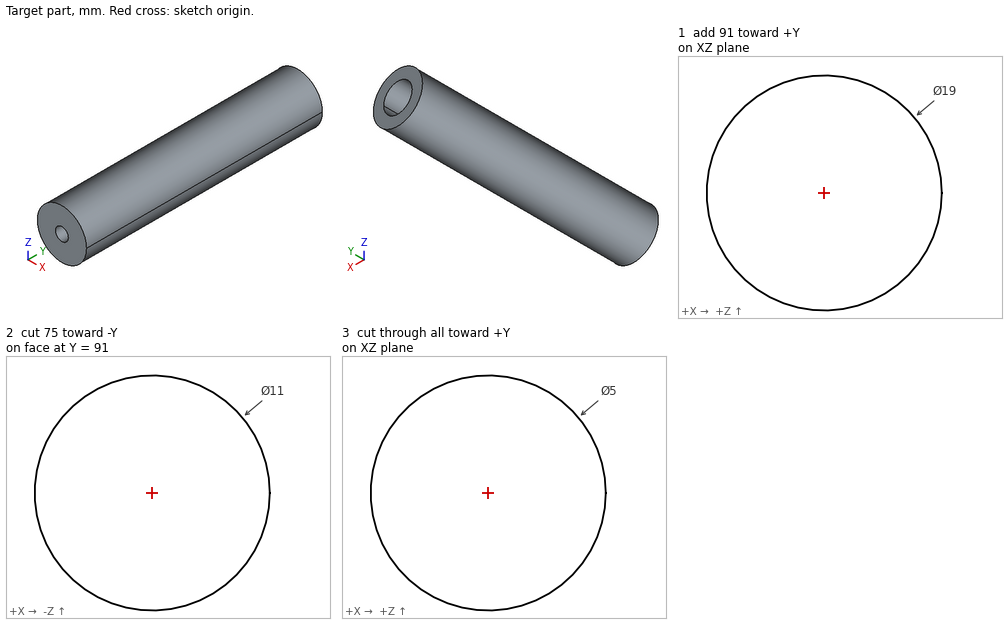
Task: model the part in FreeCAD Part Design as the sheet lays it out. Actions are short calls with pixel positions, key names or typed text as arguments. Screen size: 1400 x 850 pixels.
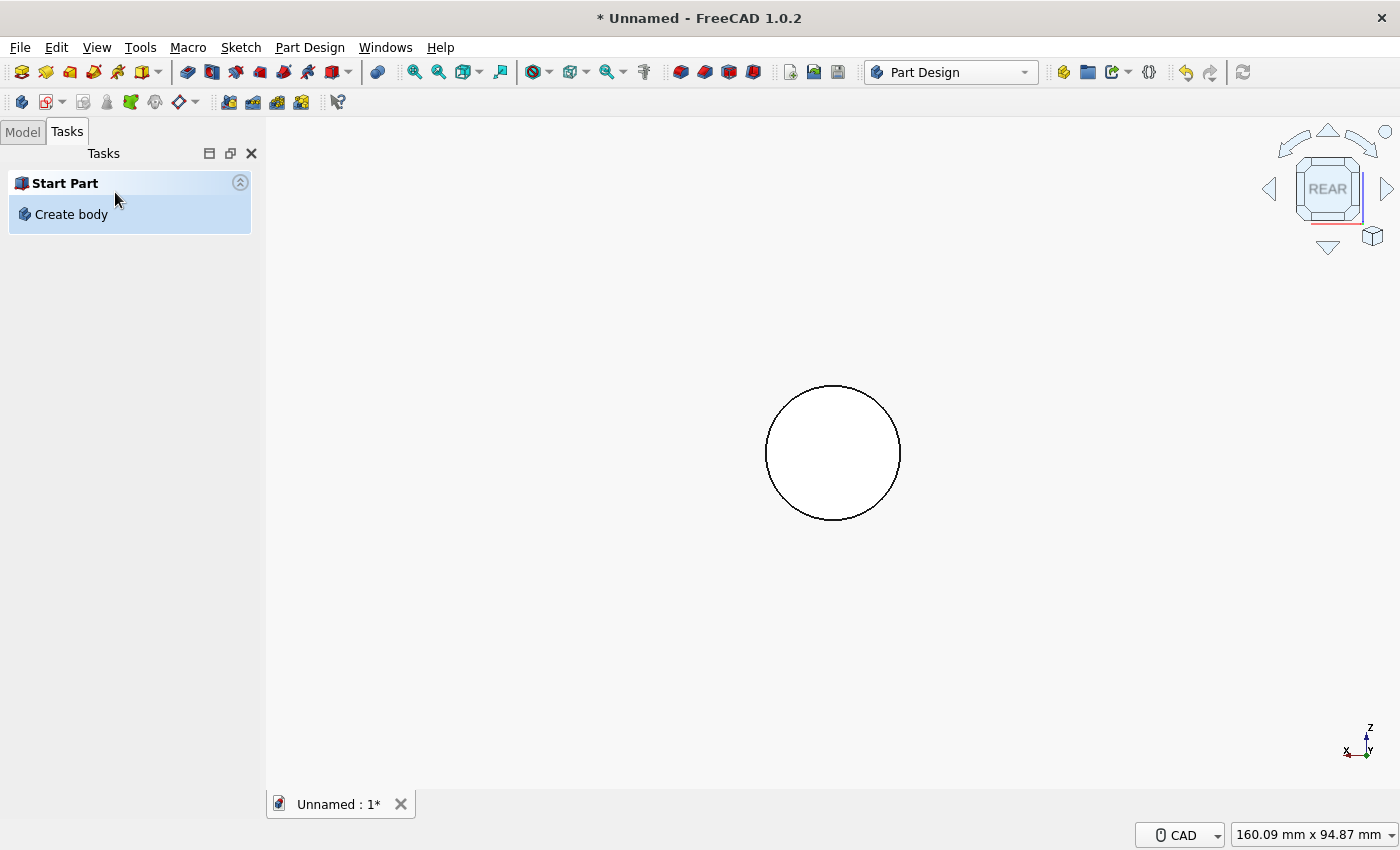
click(416, 72)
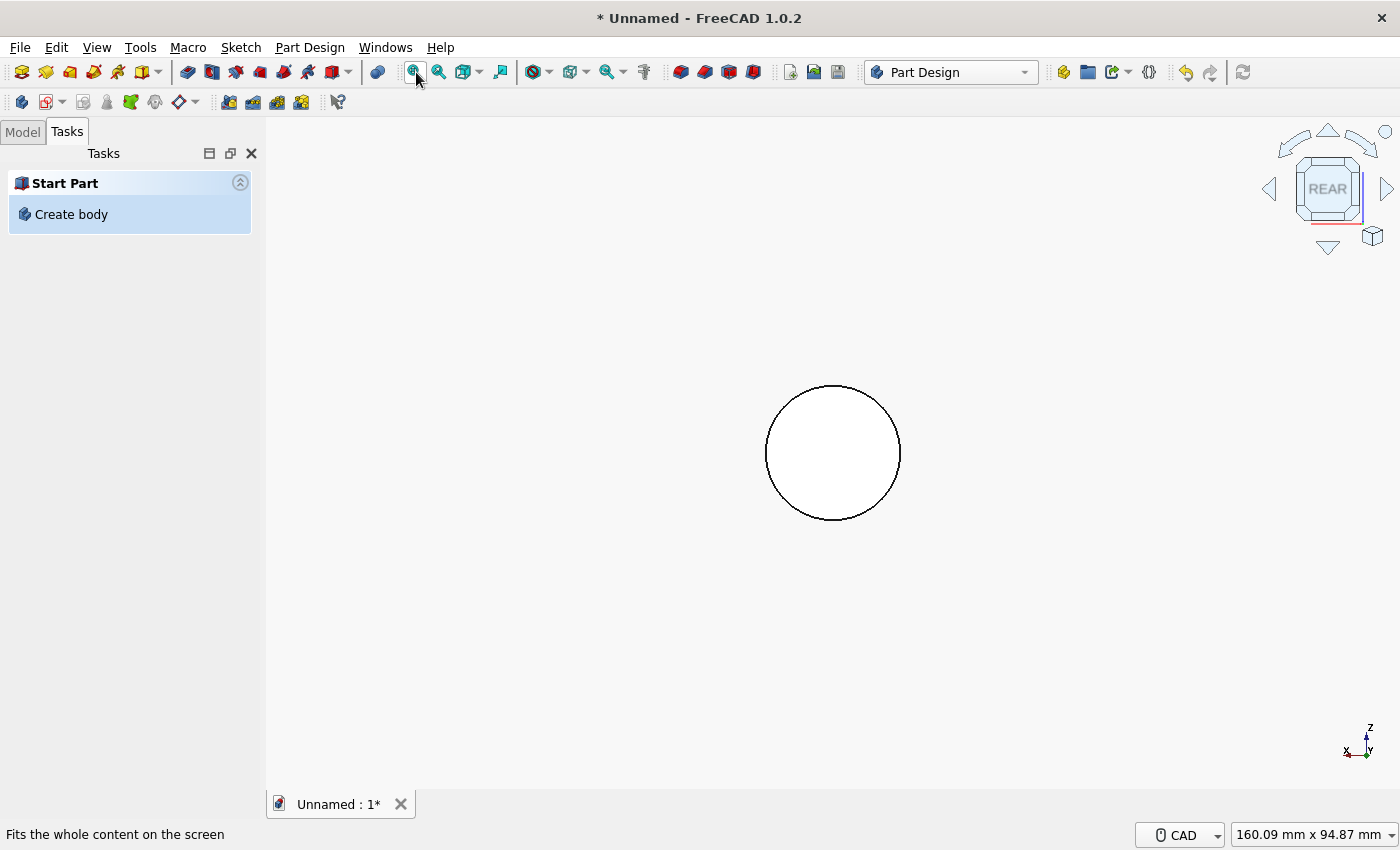
click(833, 452)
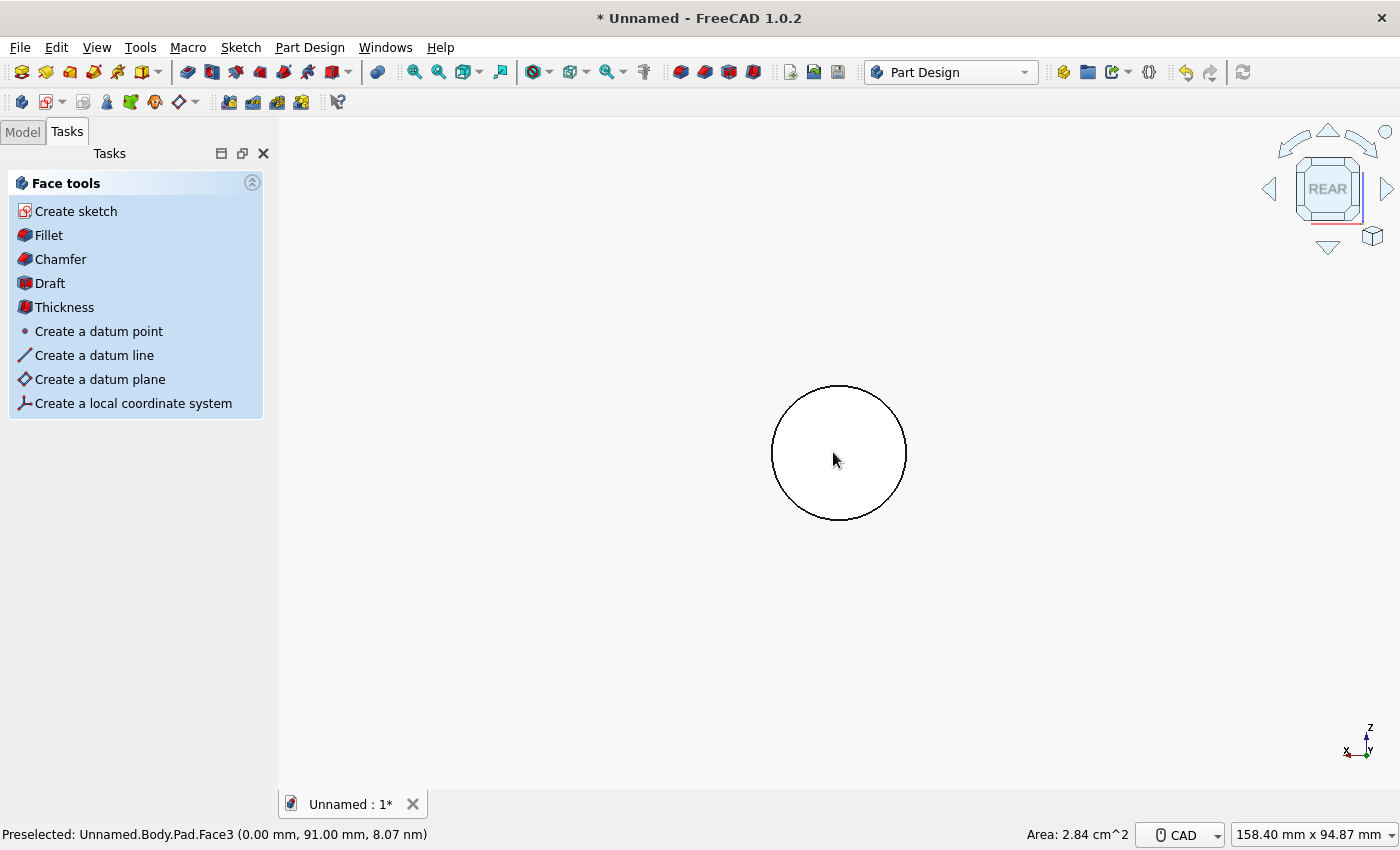
click(46, 102)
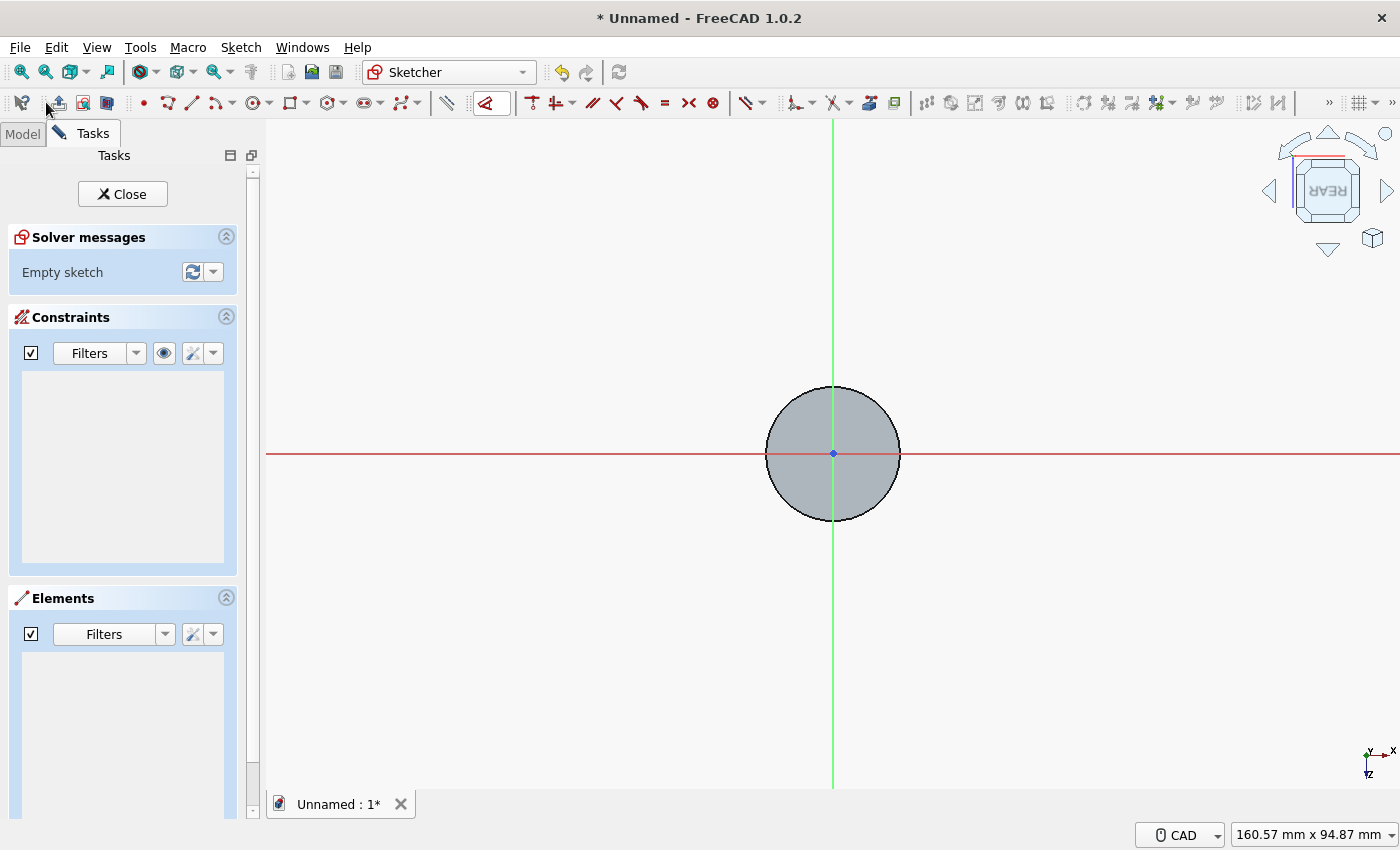
scroll(847, 454, up, 9)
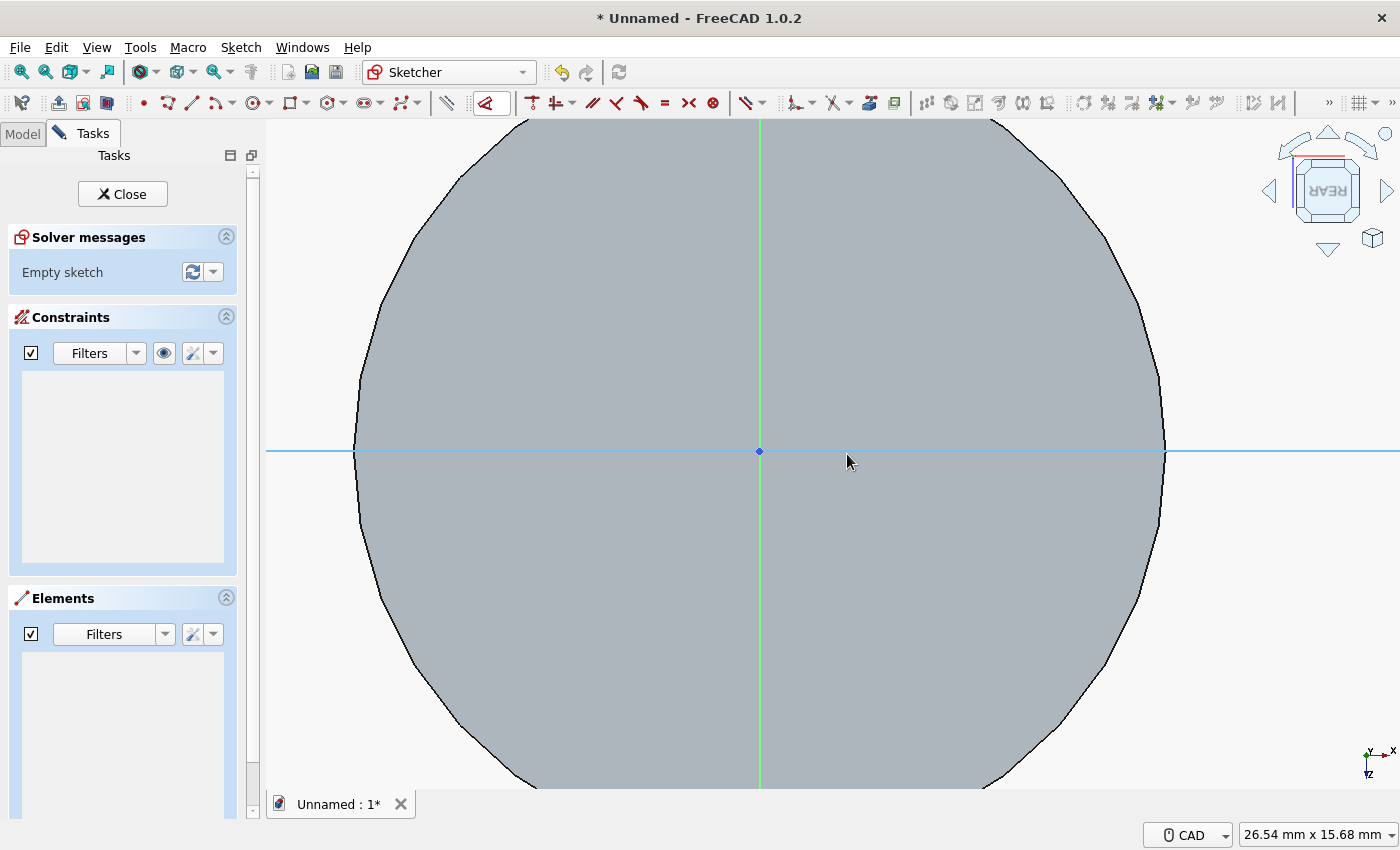
click(254, 104)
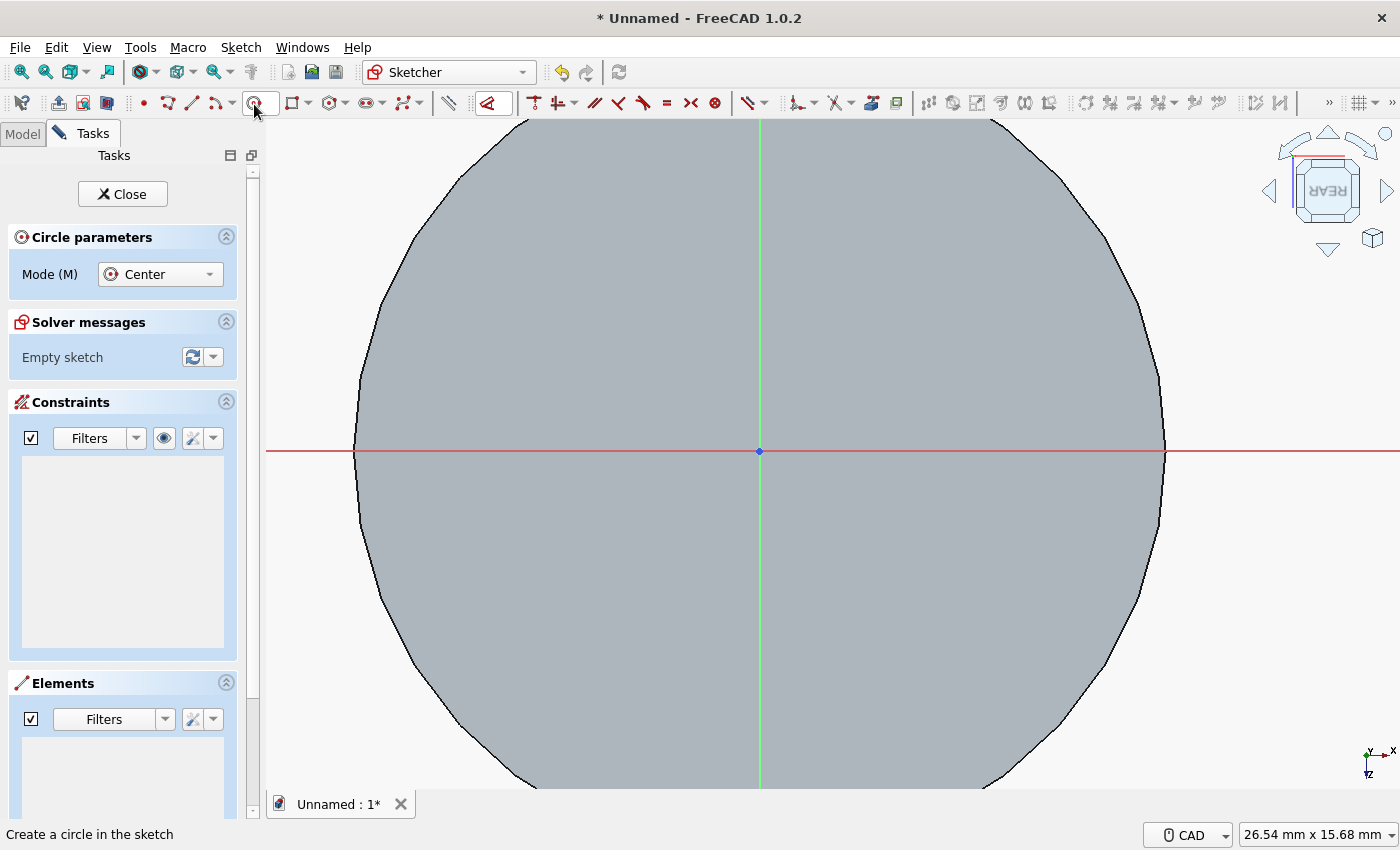
click(760, 451)
click(926, 285)
key(Escape)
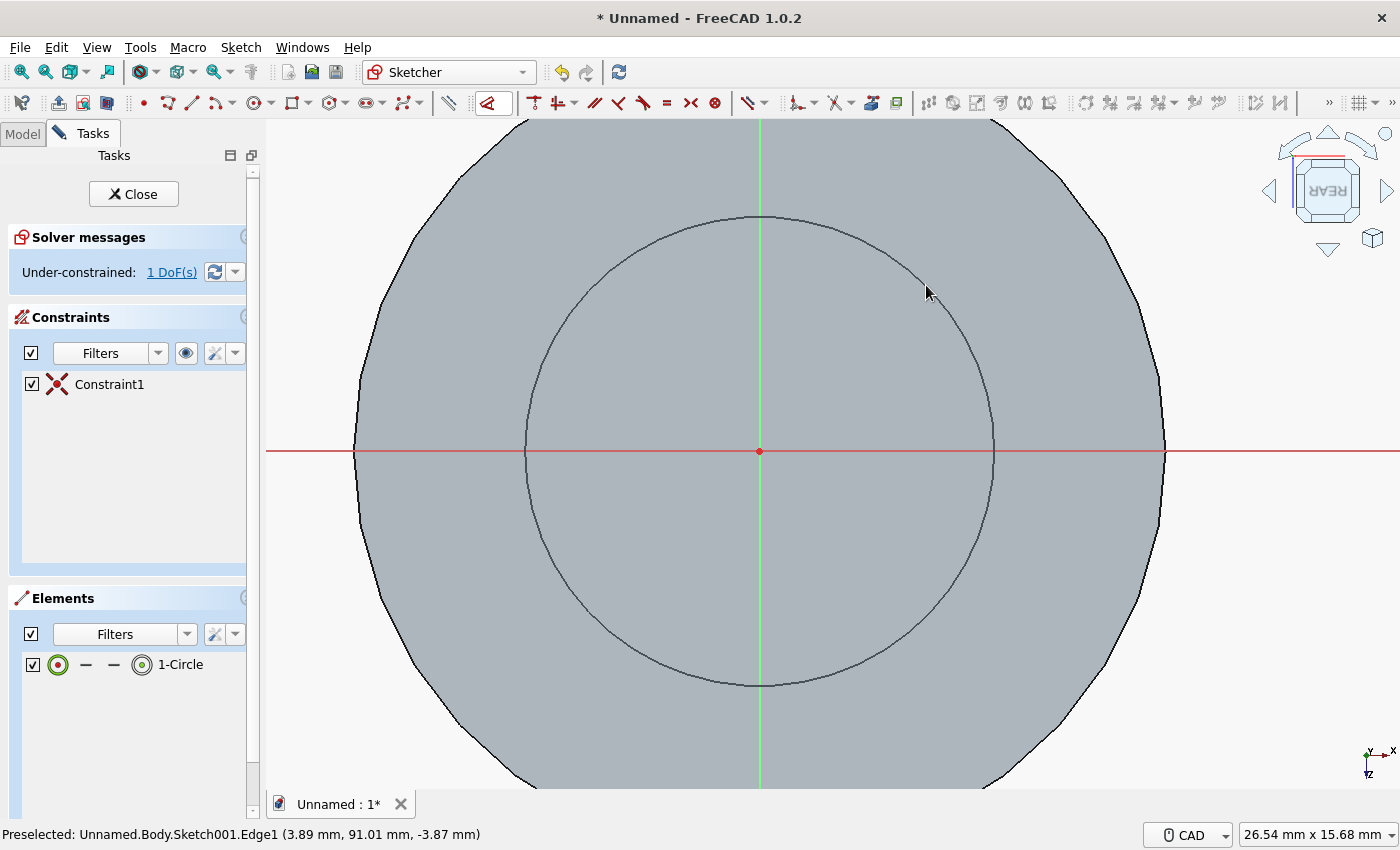
click(925, 285)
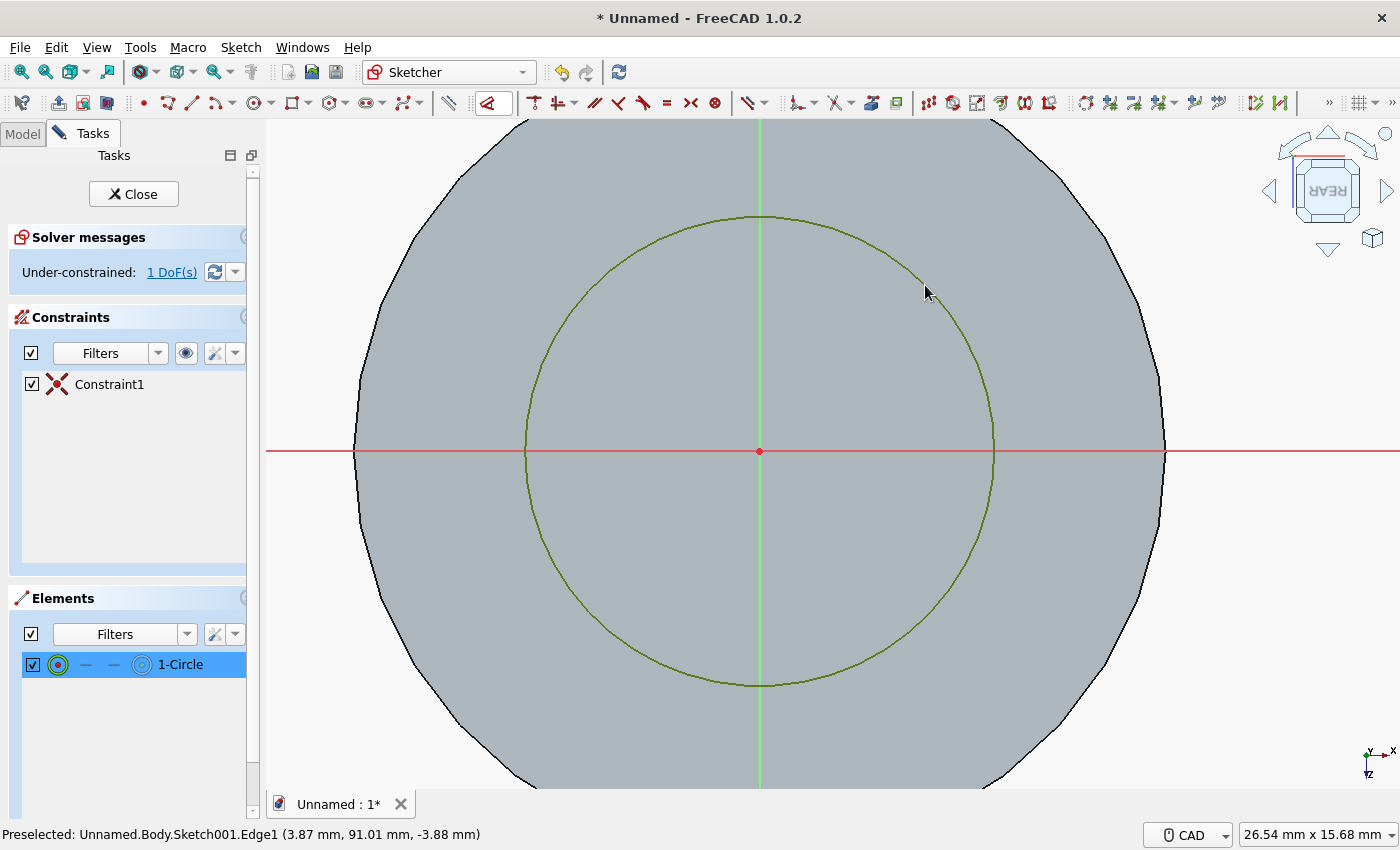
key(k)
key(o)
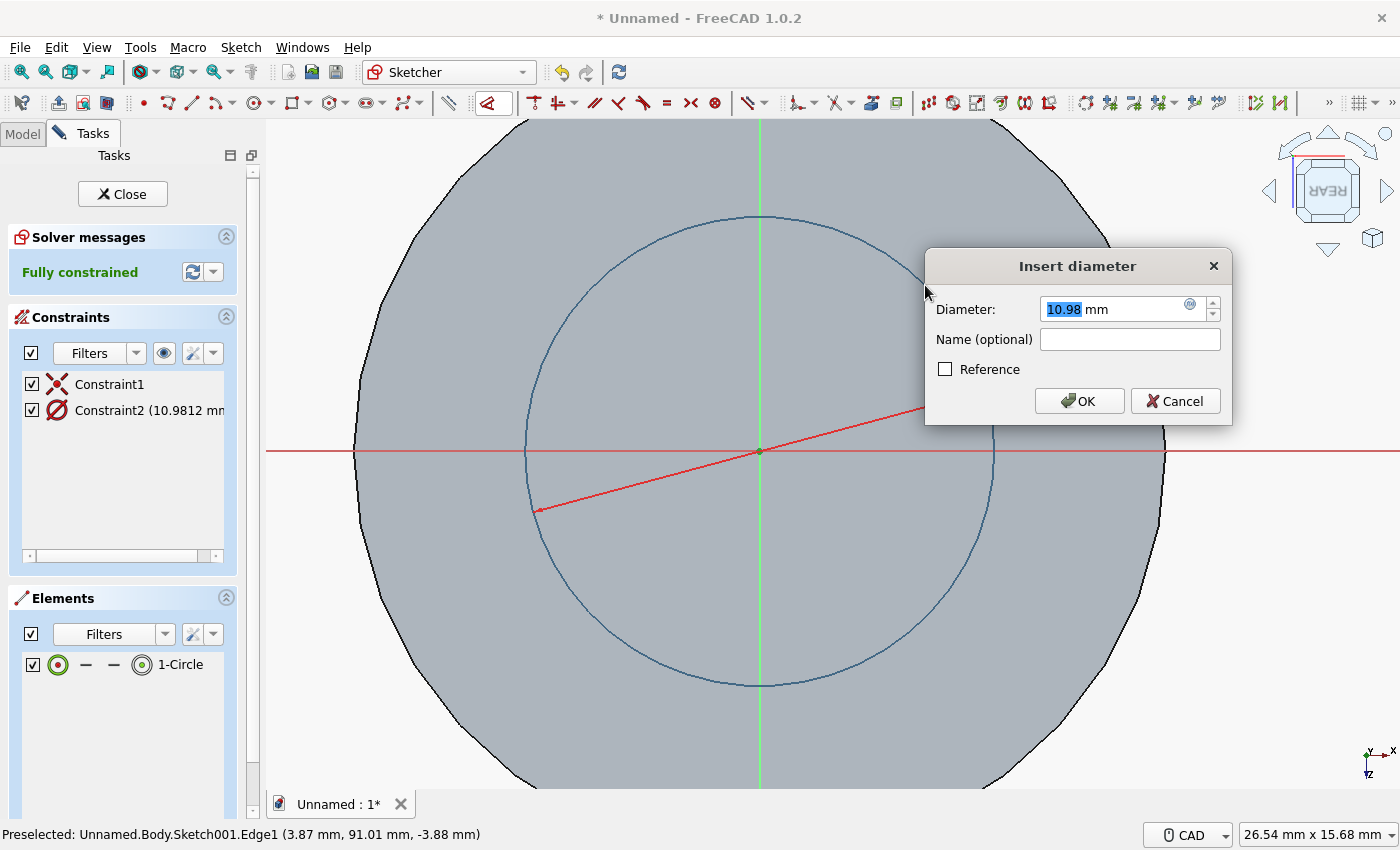
text(11)
key(Return)